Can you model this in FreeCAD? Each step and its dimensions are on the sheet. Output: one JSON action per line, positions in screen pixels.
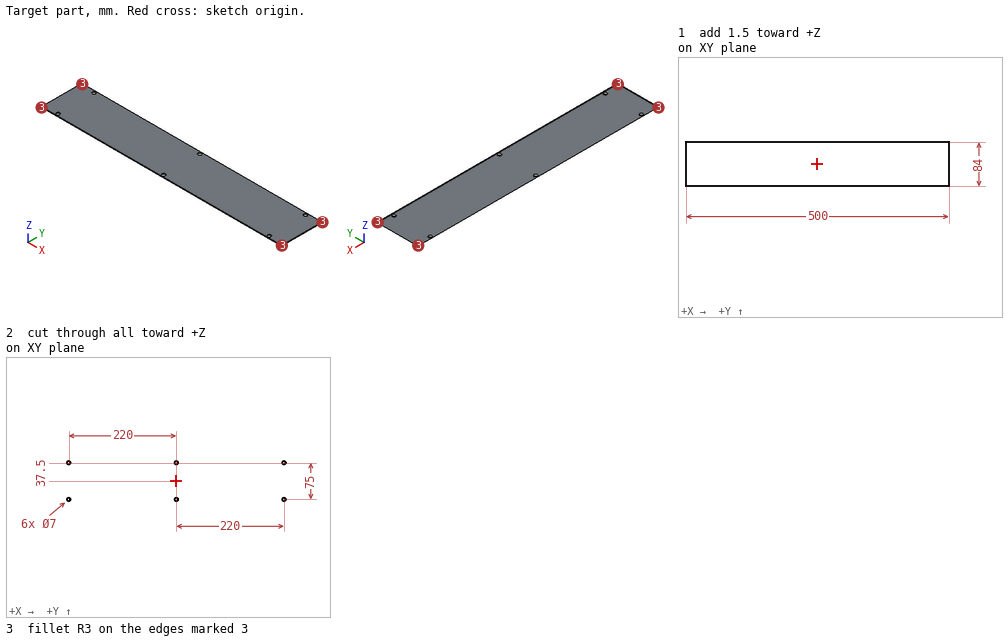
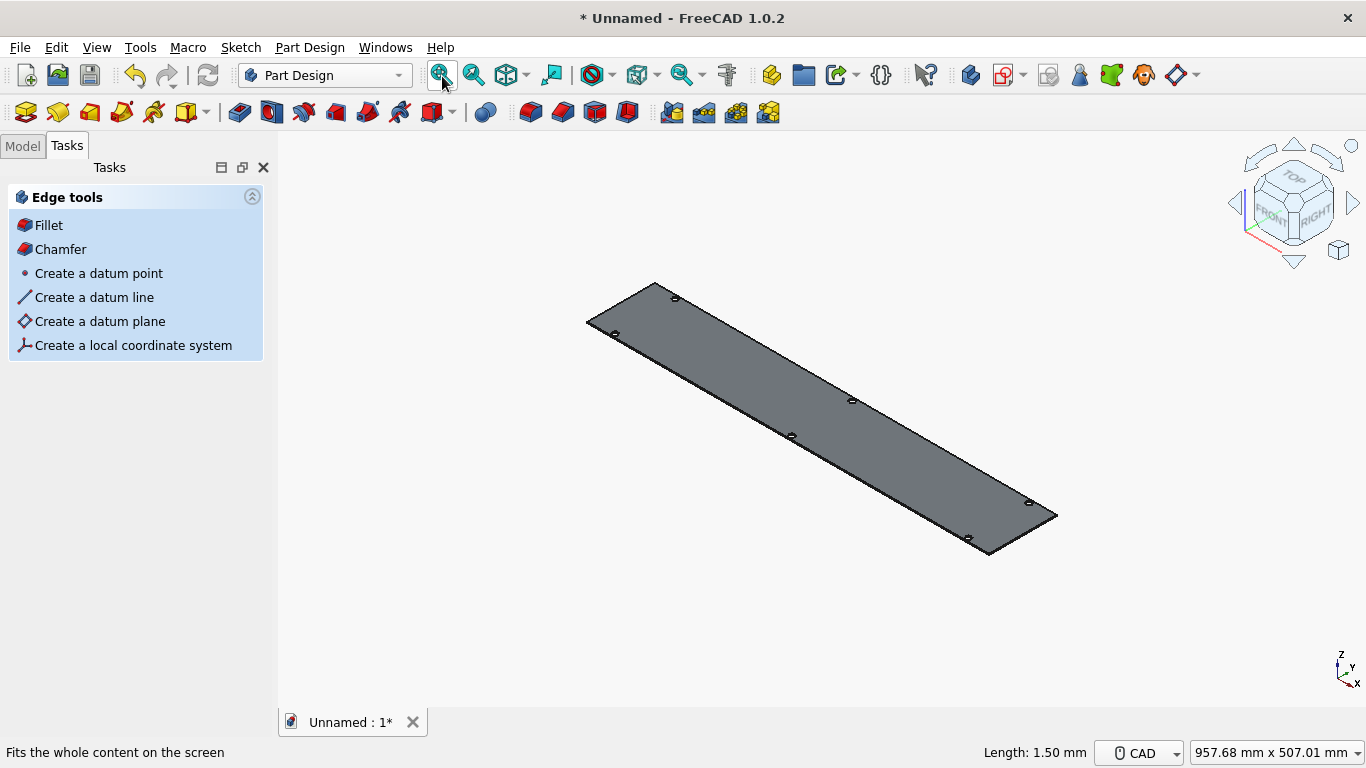
{"action": "key", "text": "2"}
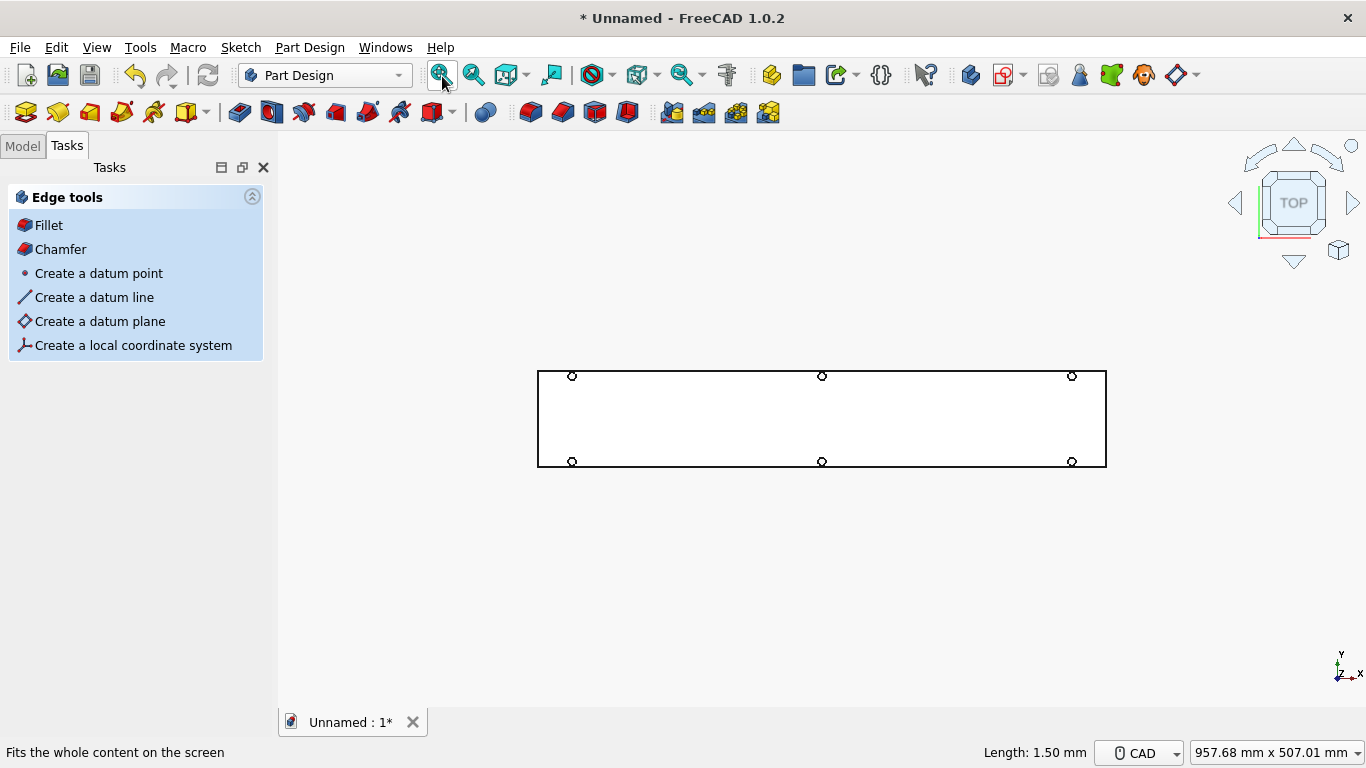
{"action": "scroll", "coordinate": [538, 466], "scroll_direction": "up", "scroll_amount": 15}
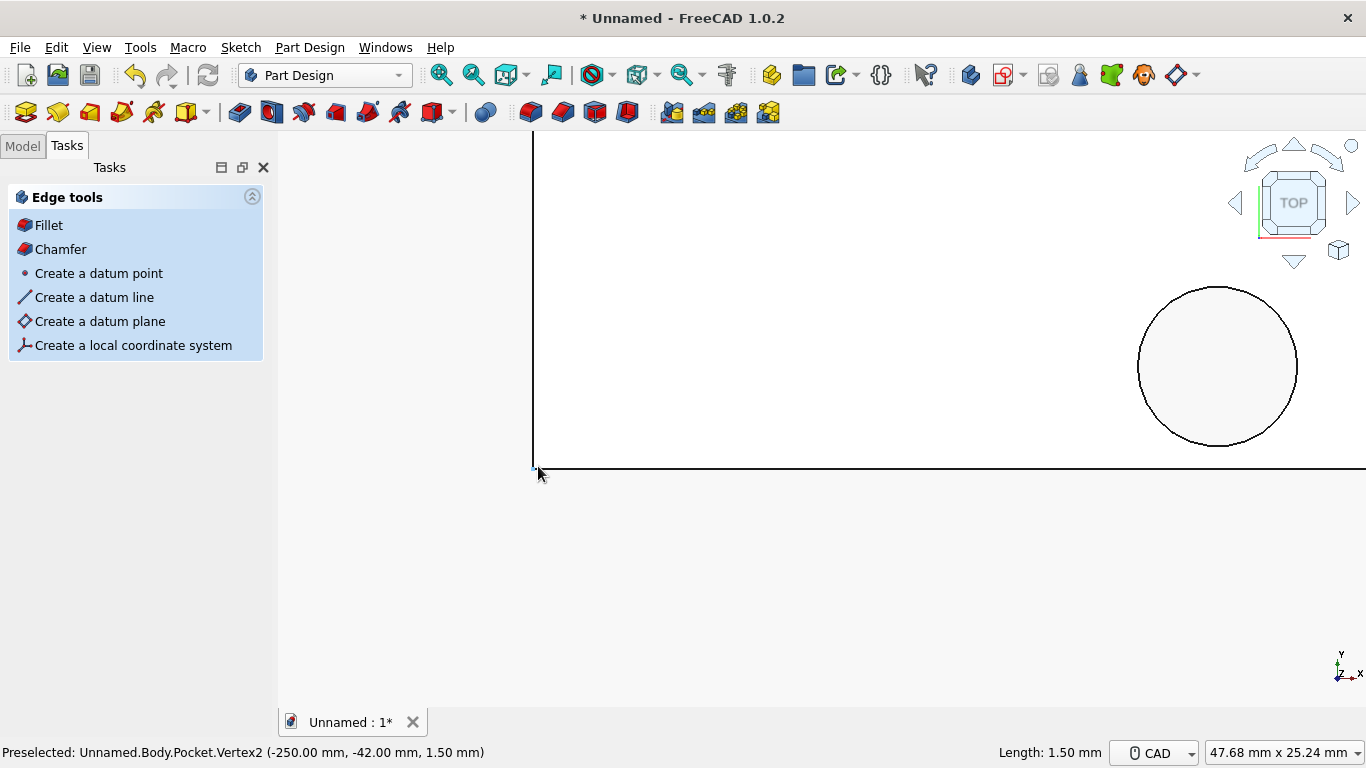
{"action": "key", "text": "v f"}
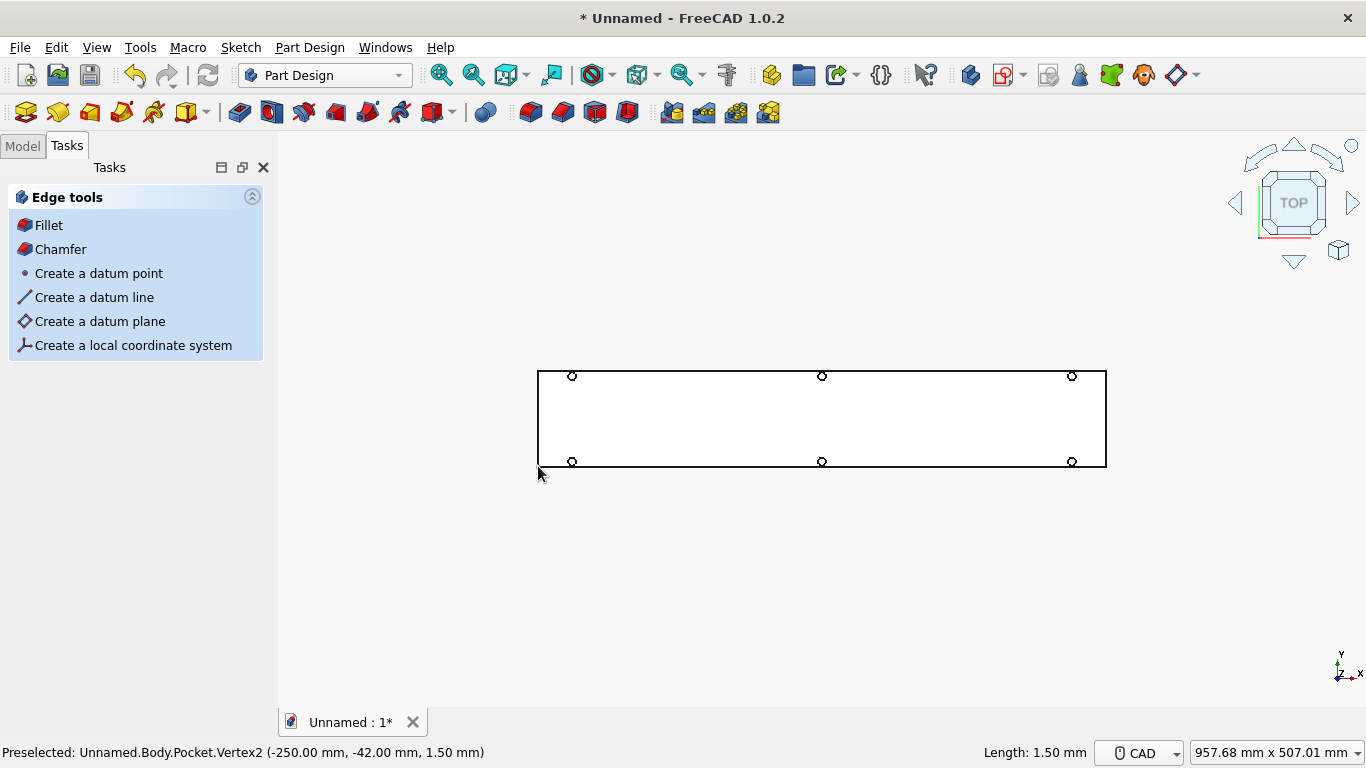
{"action": "key", "text": "1"}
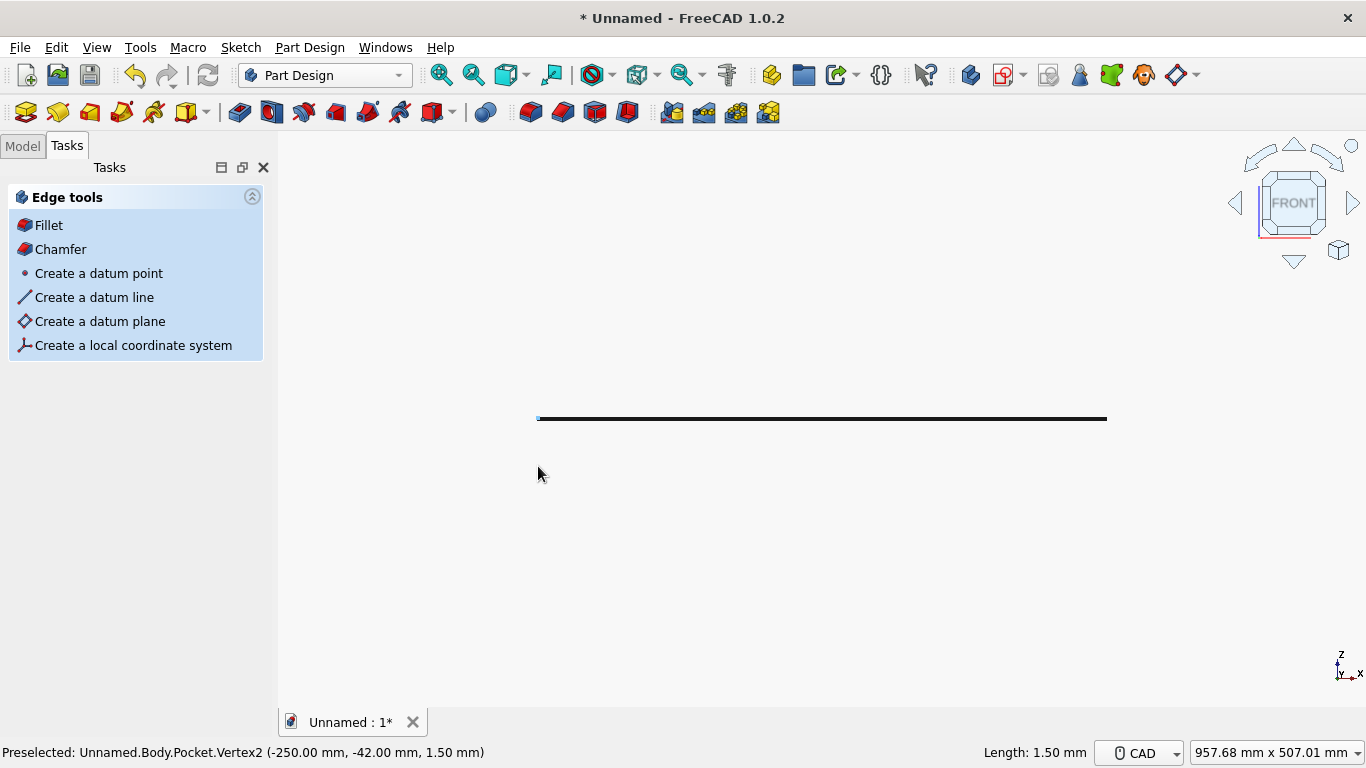
{"action": "scroll", "coordinate": [538, 418], "scroll_direction": "up", "scroll_amount": 15}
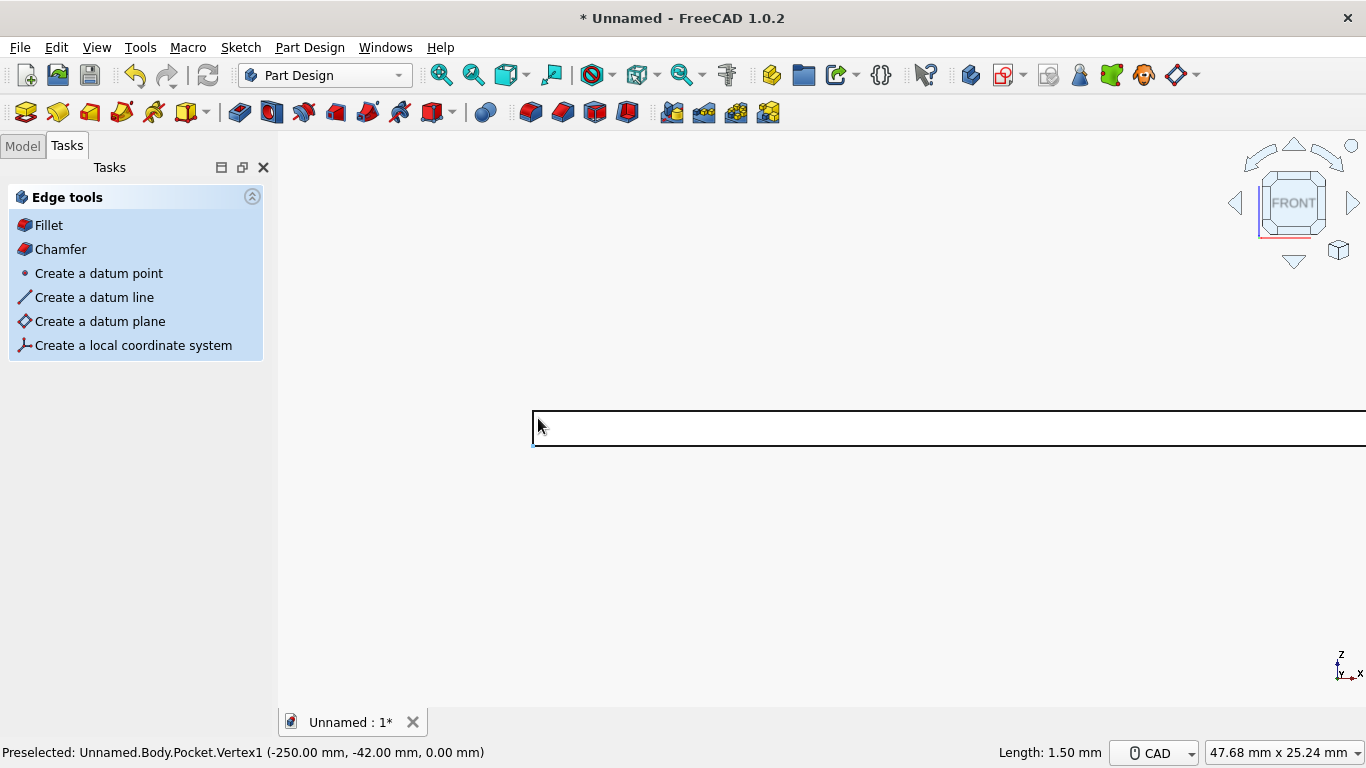
{"action": "left_click", "coordinate": [533, 428], "text": "ctrl"}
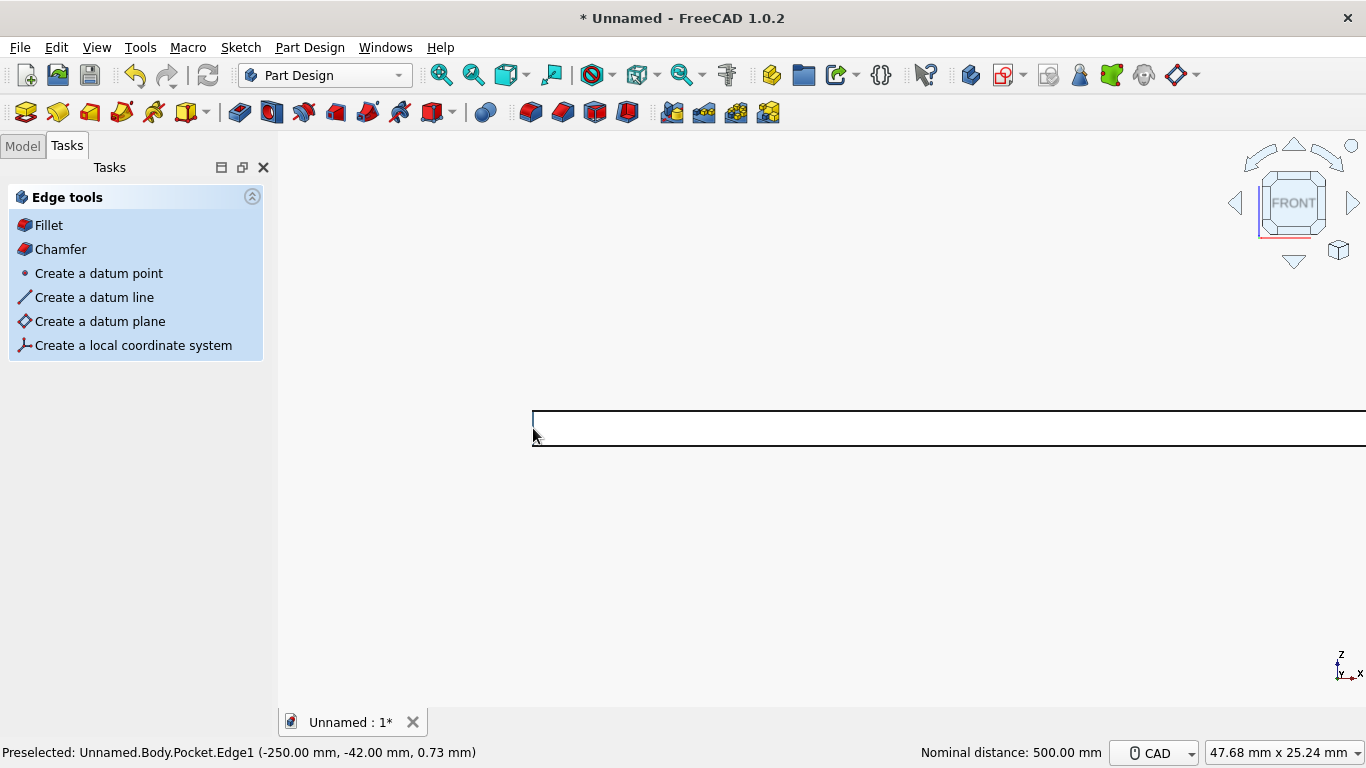
{"action": "key", "text": "v f"}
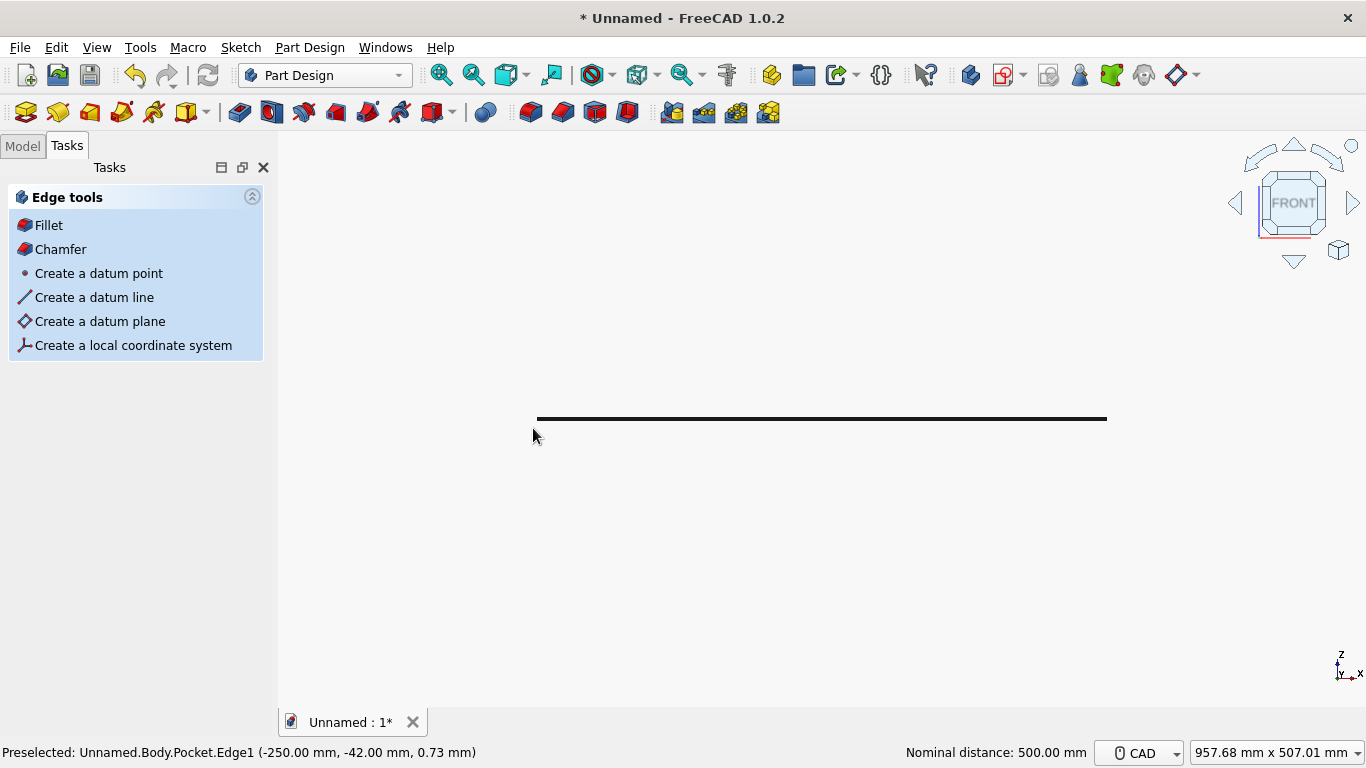
{"action": "key", "text": "3"}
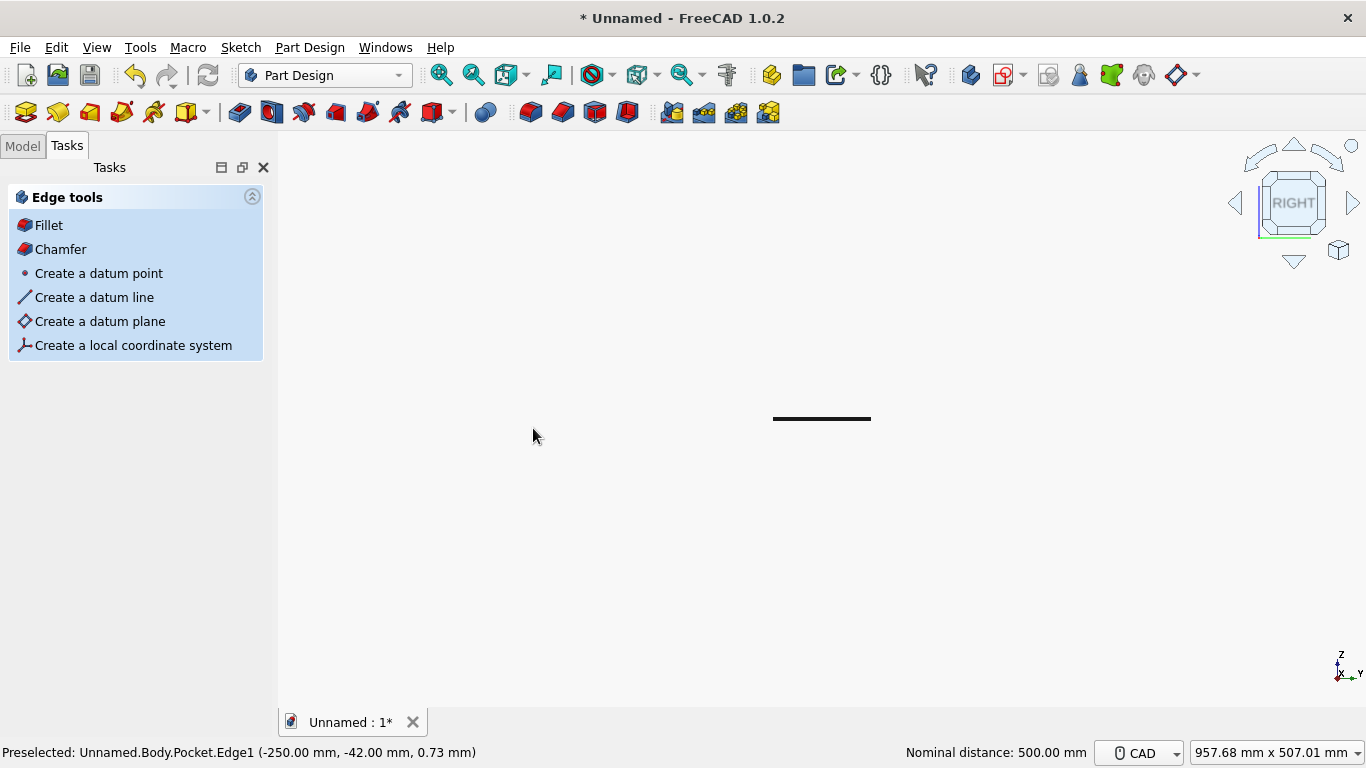
{"action": "left_click", "coordinate": [442, 76]}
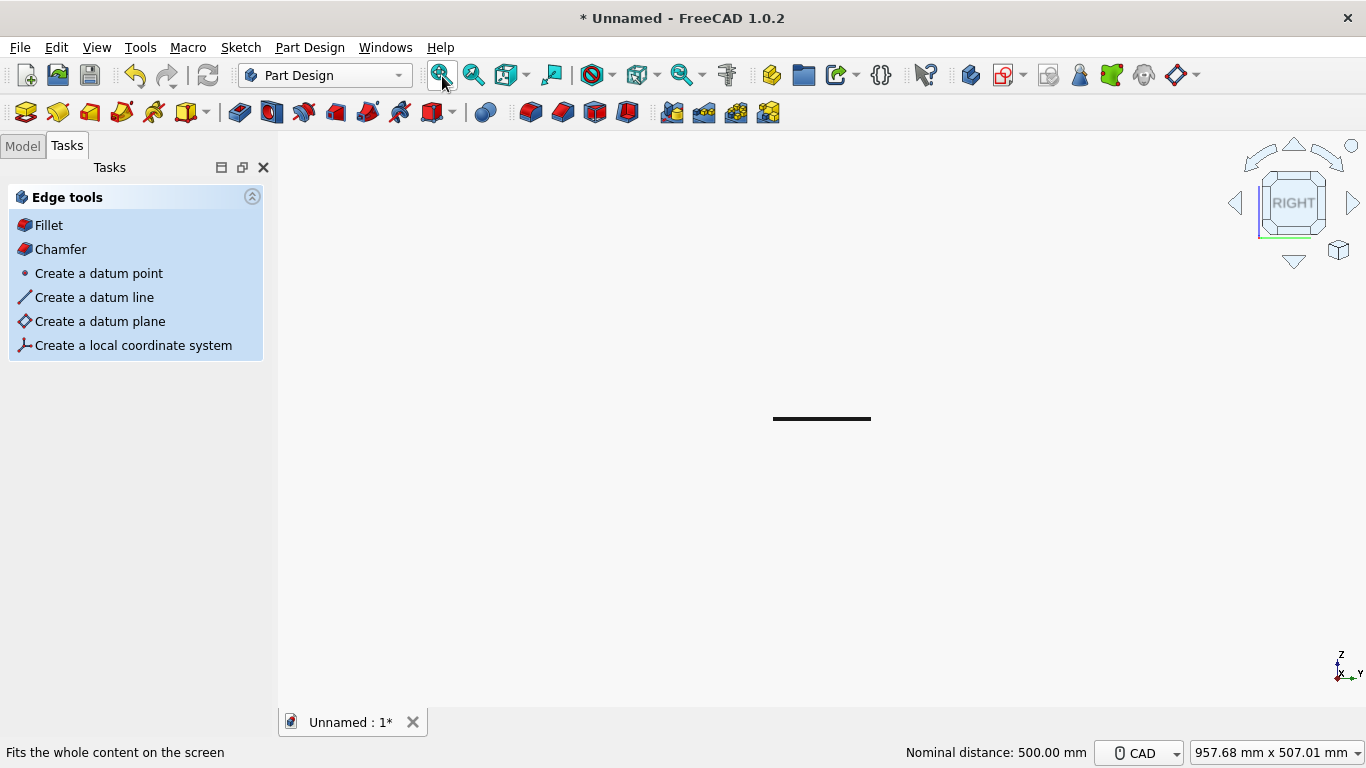
{"action": "scroll", "coordinate": [870, 418], "scroll_direction": "up", "scroll_amount": 15}